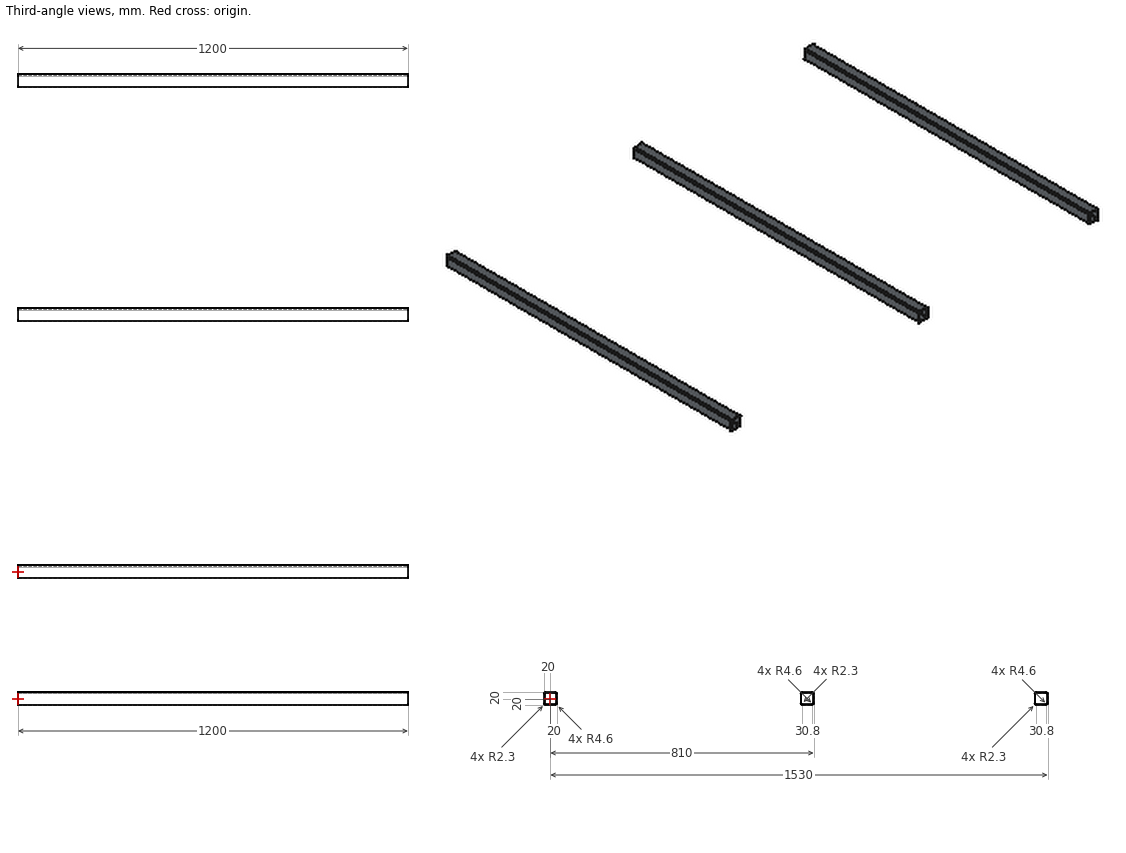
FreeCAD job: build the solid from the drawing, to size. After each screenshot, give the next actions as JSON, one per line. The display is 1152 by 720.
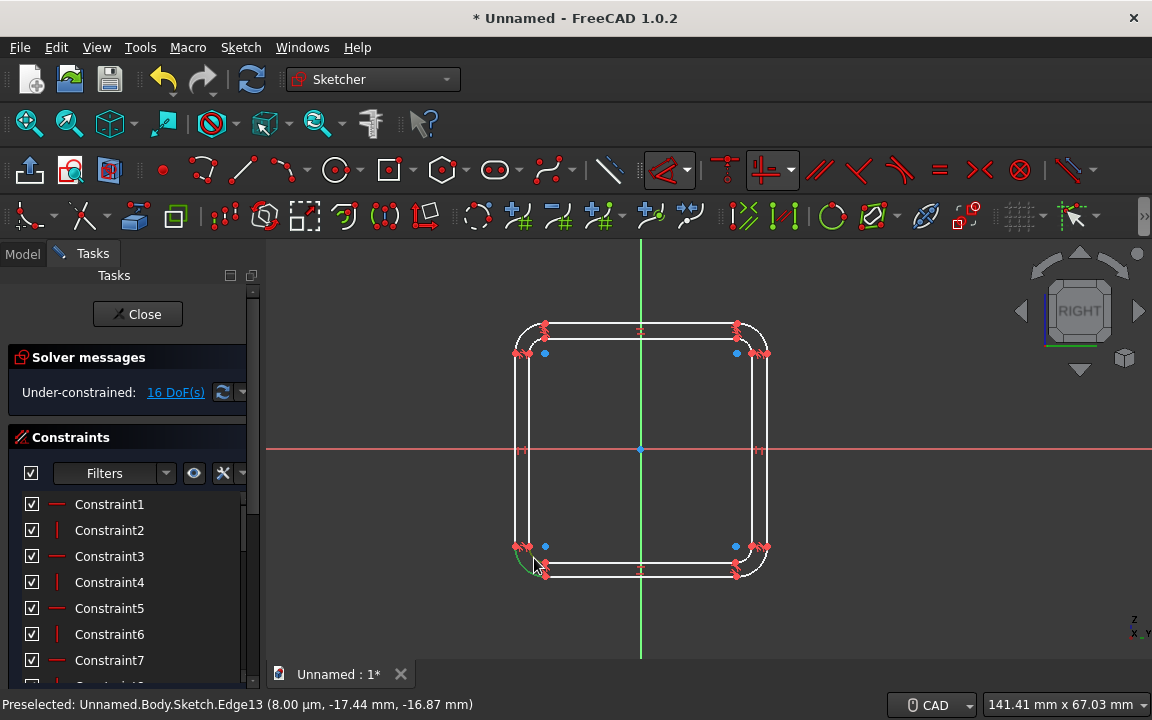
{"action": "left_click", "coordinate": [726, 170]}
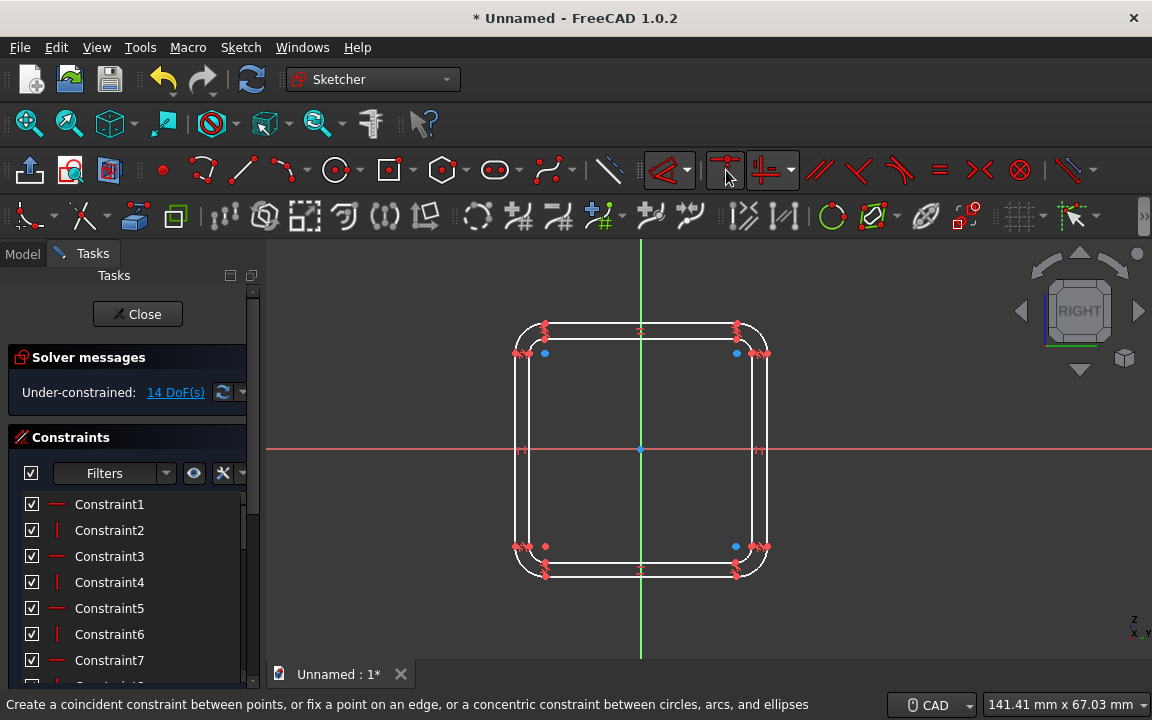
{"action": "left_click", "coordinate": [532, 327]}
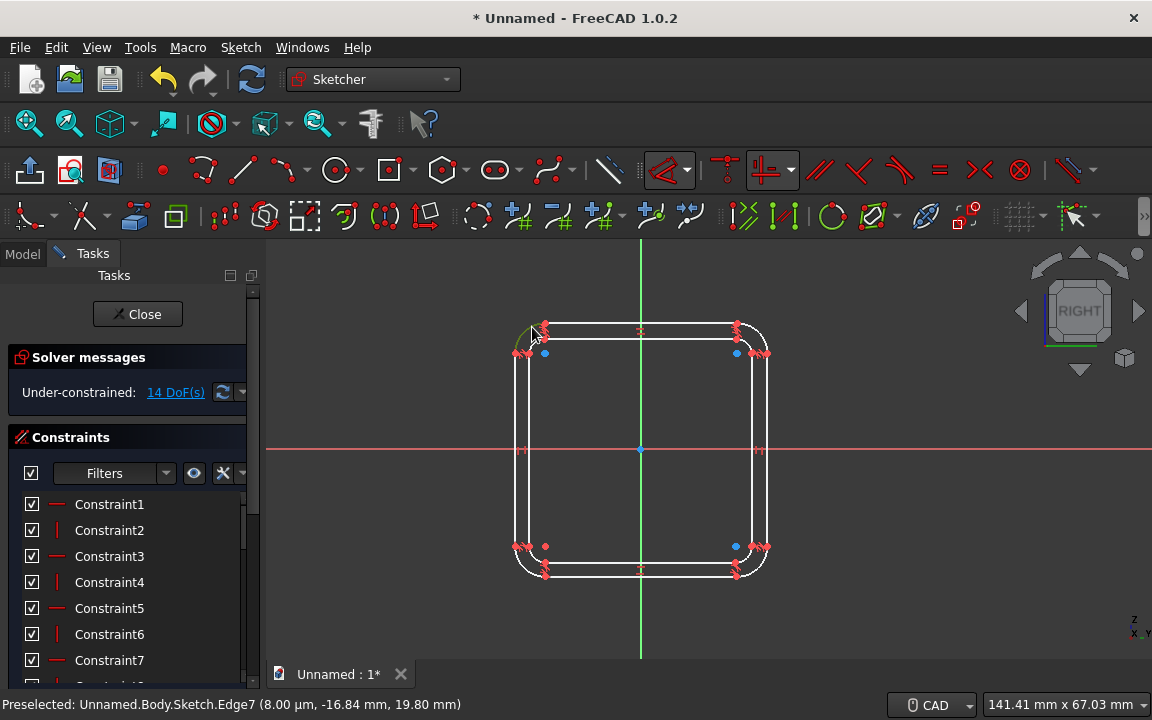
{"action": "scroll", "coordinate": [534, 343], "scroll_direction": "up", "scroll_amount": 2}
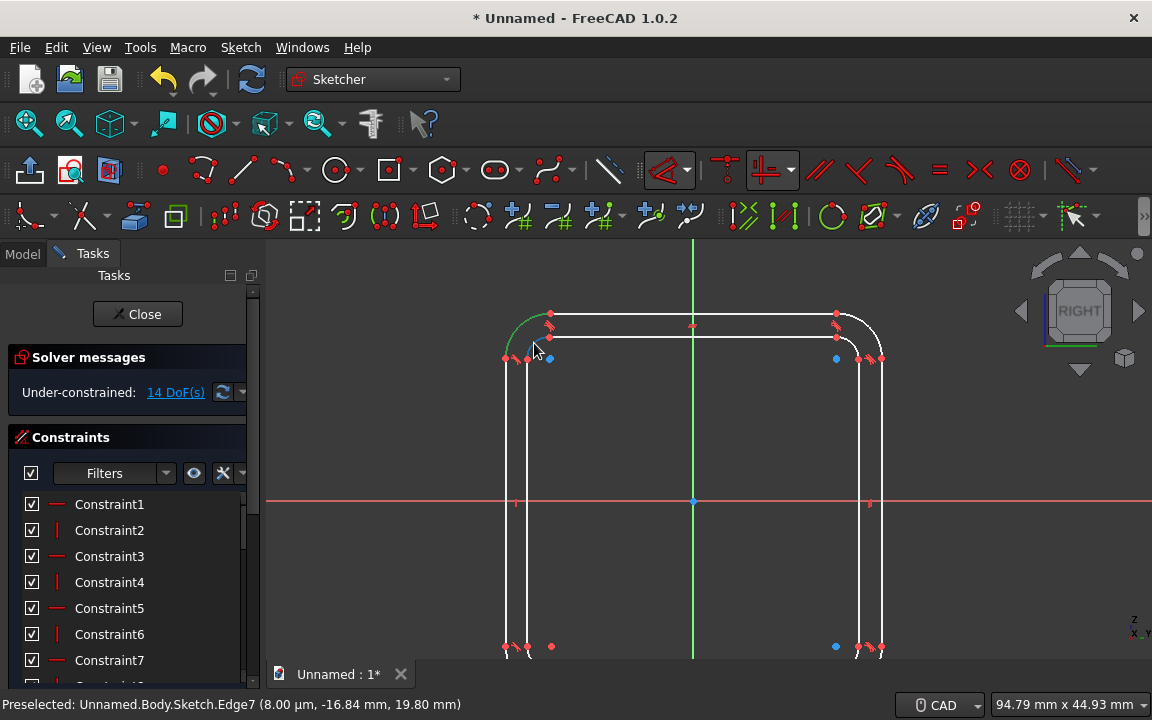
{"action": "left_click", "coordinate": [534, 344]}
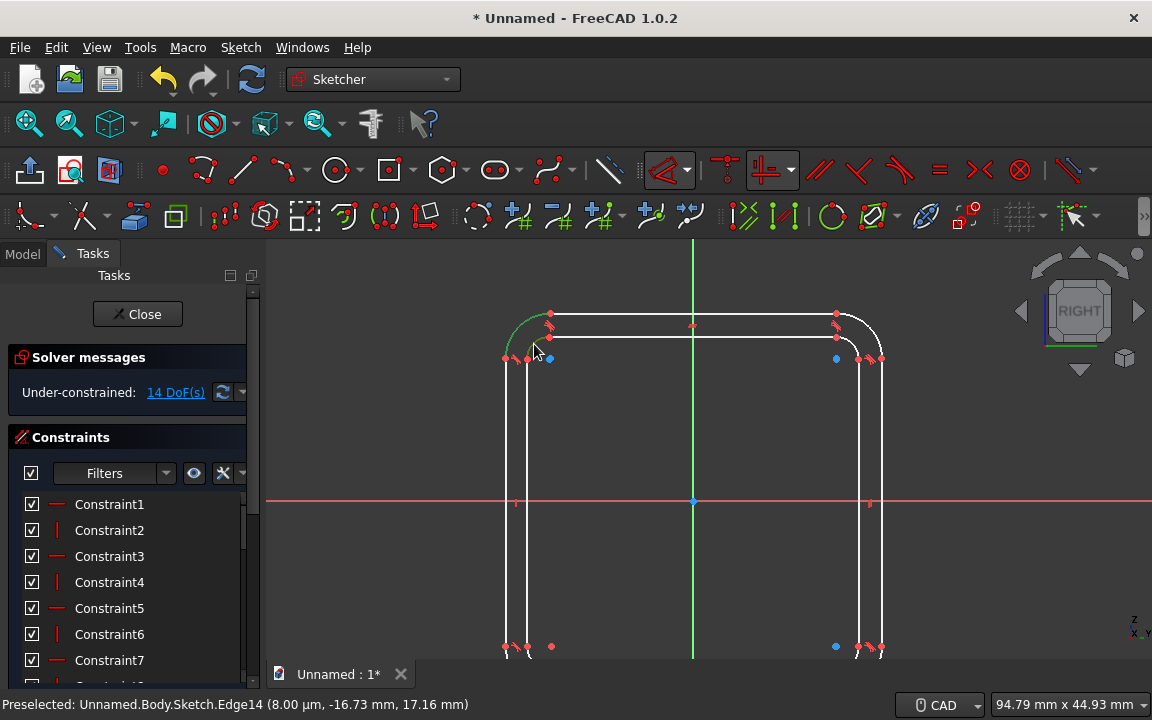
{"action": "left_click", "coordinate": [726, 170]}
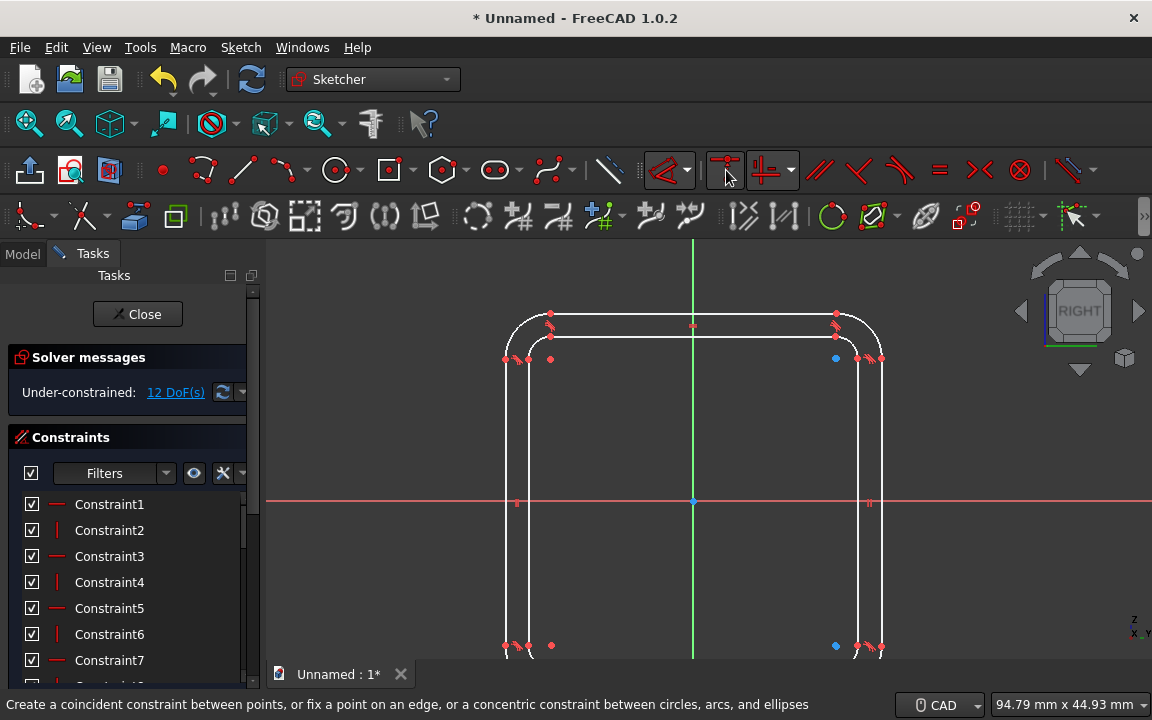
{"action": "left_click", "coordinate": [877, 338]}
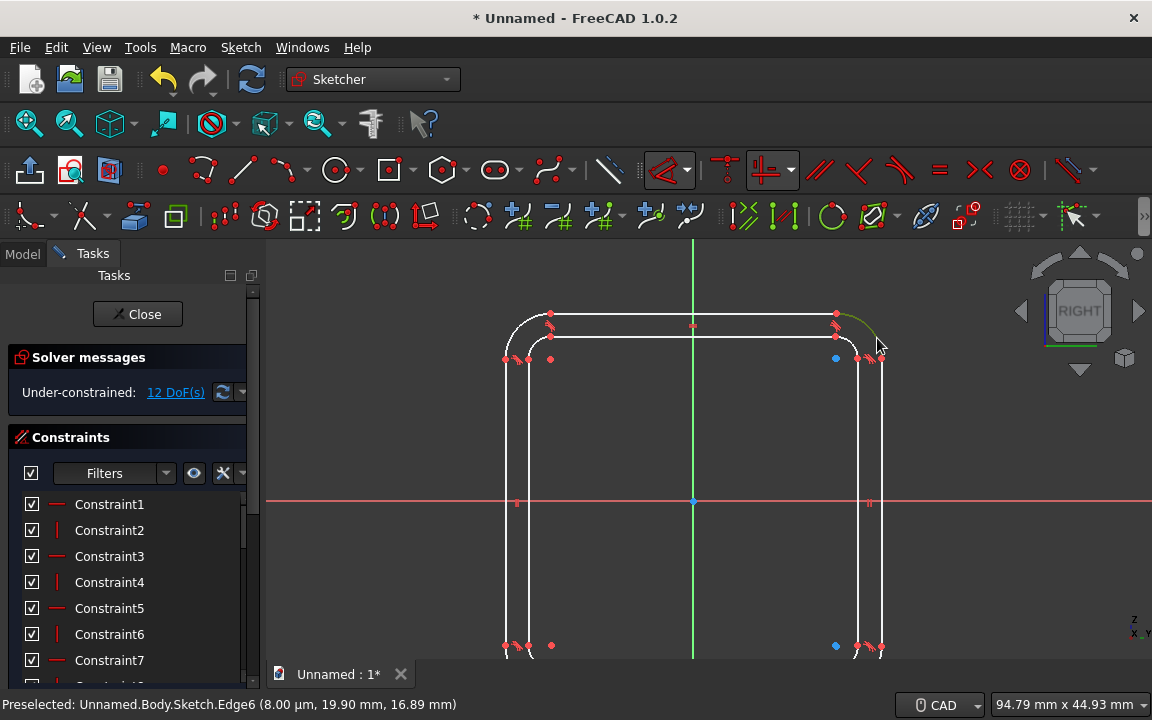
{"action": "scroll", "coordinate": [856, 349], "scroll_direction": "up", "scroll_amount": 2}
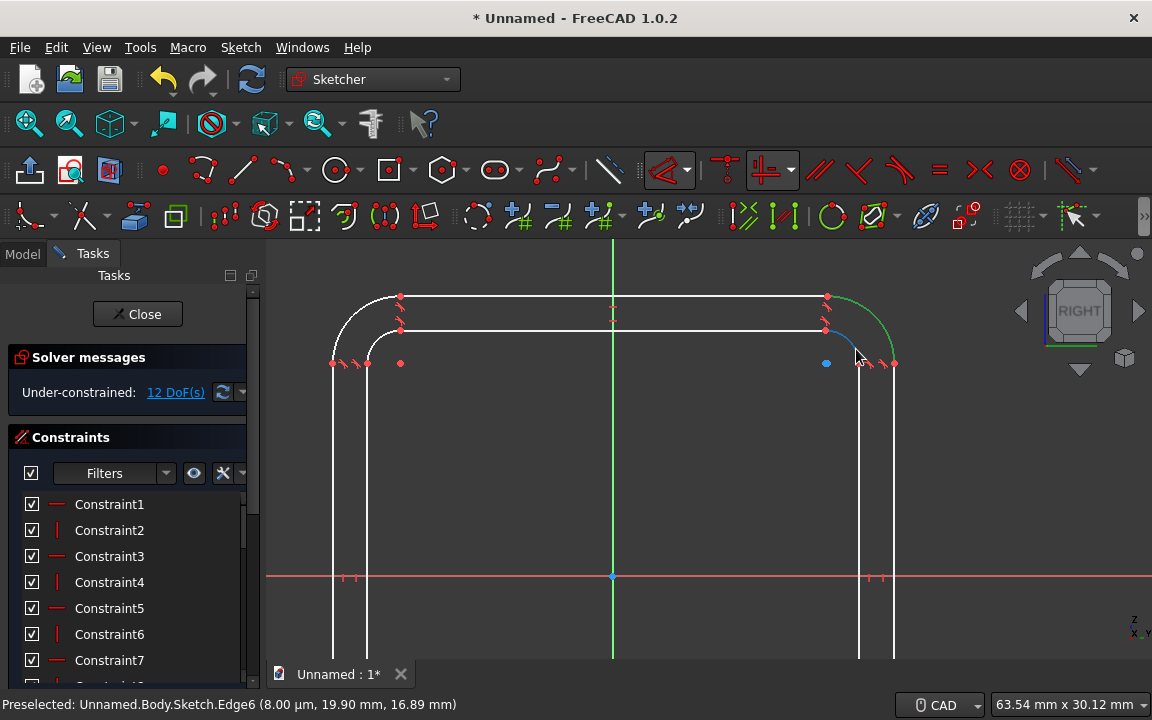
{"action": "left_click", "coordinate": [855, 349]}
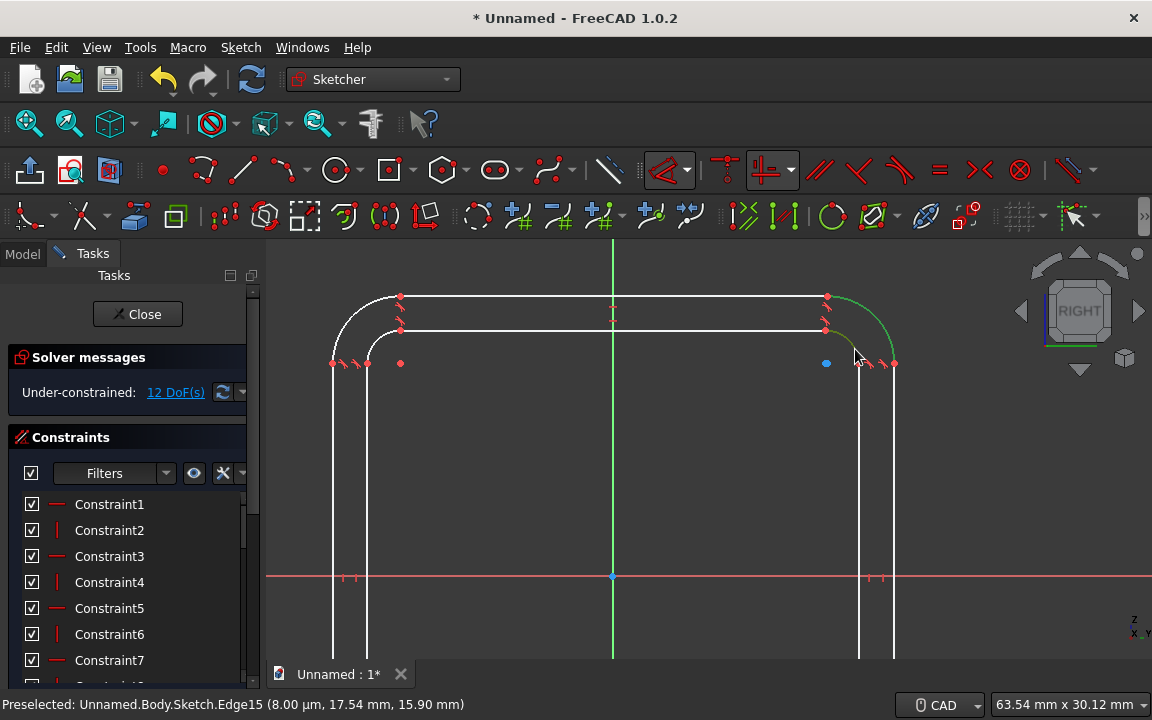
{"action": "key", "text": "c"}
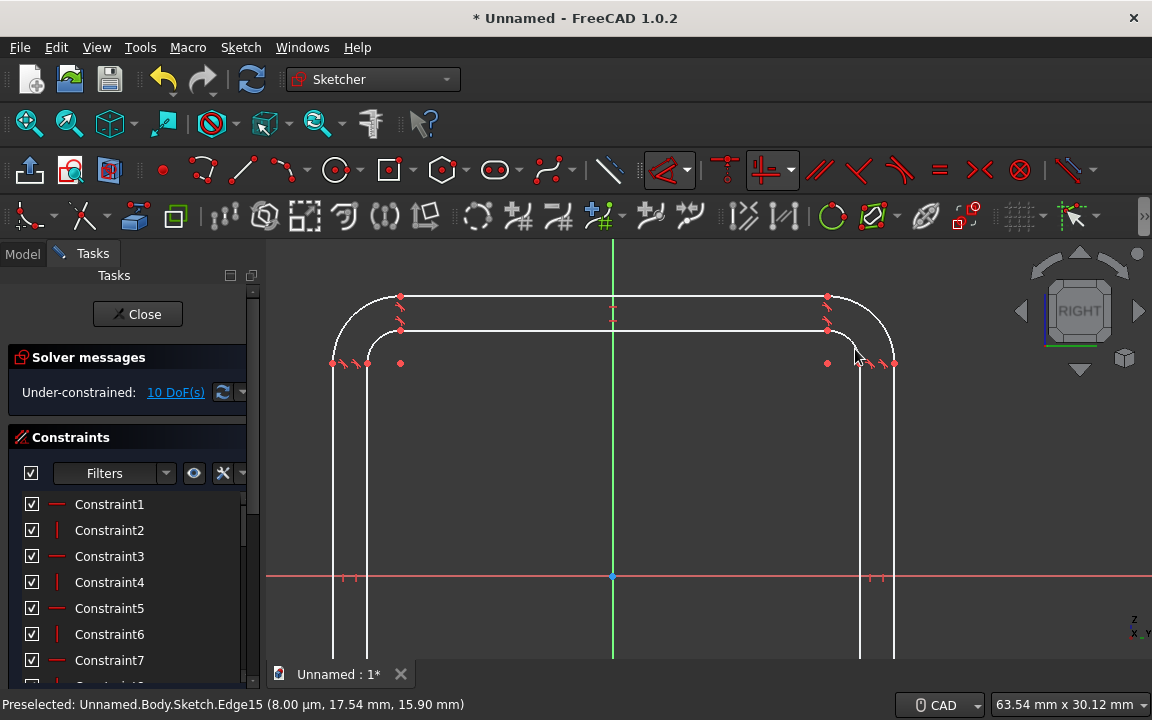
{"action": "scroll", "coordinate": [663, 345], "scroll_direction": "down", "scroll_amount": 4}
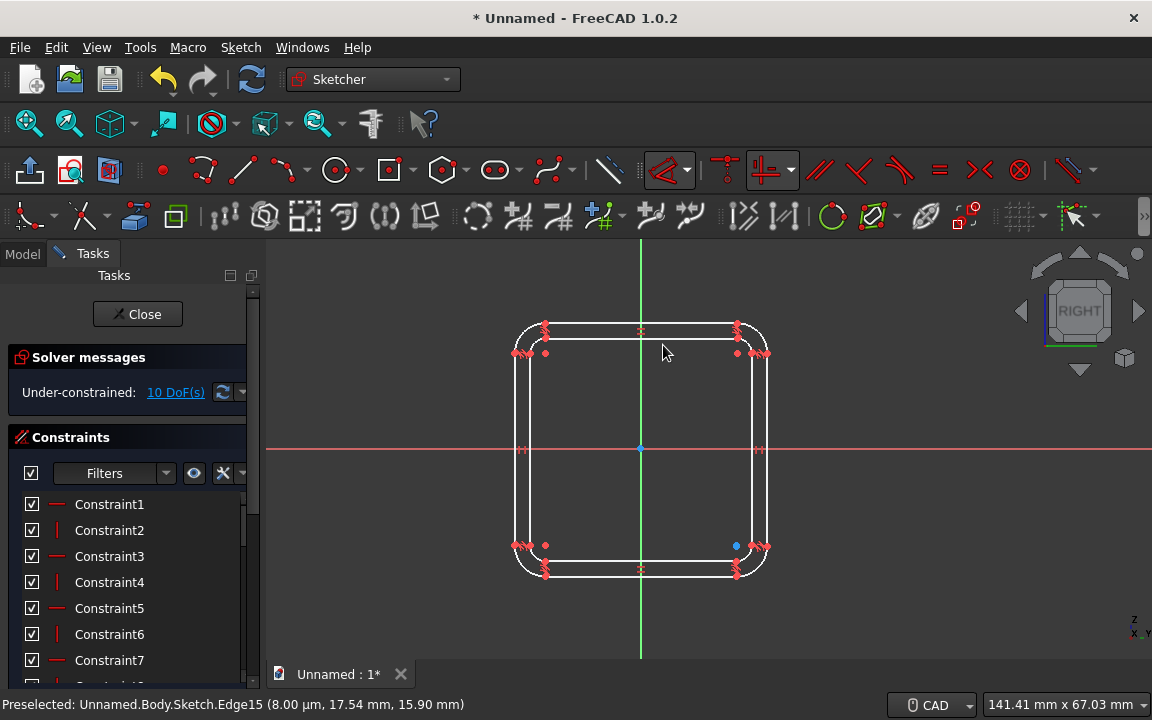
{"action": "left_click", "coordinate": [751, 573]}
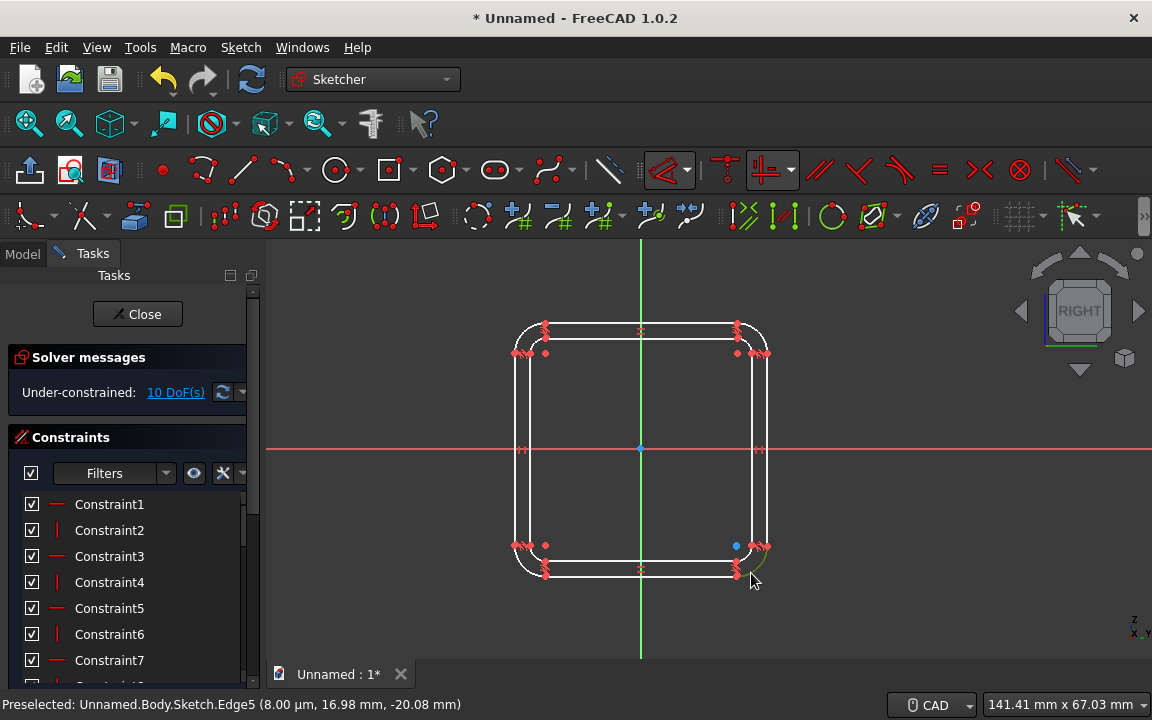
{"action": "left_click", "coordinate": [764, 340]}